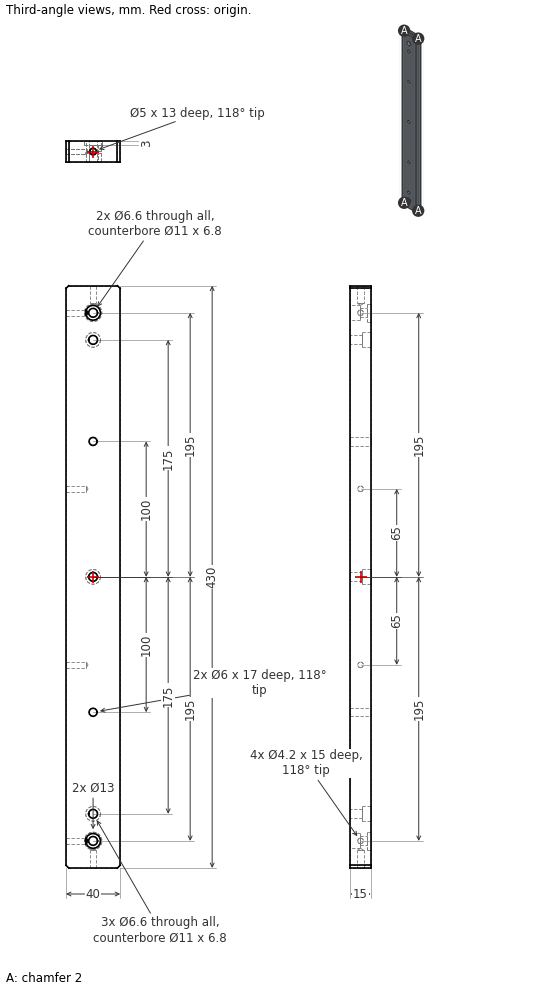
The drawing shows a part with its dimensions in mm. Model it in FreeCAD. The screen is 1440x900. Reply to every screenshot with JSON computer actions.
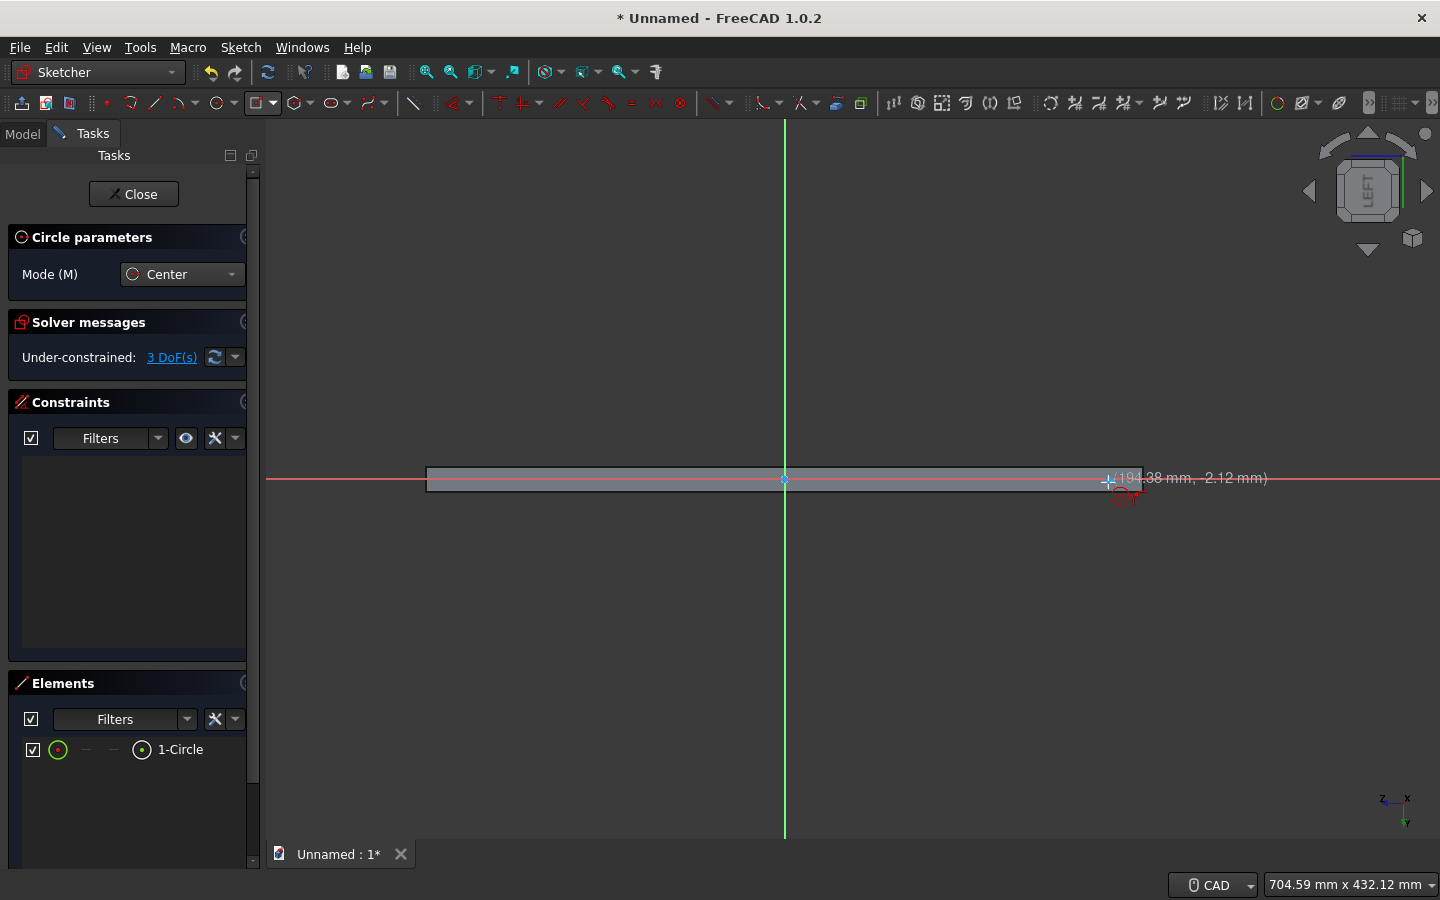
{"action": "scroll", "coordinate": [460, 479], "scroll_direction": "up", "scroll_amount": 10}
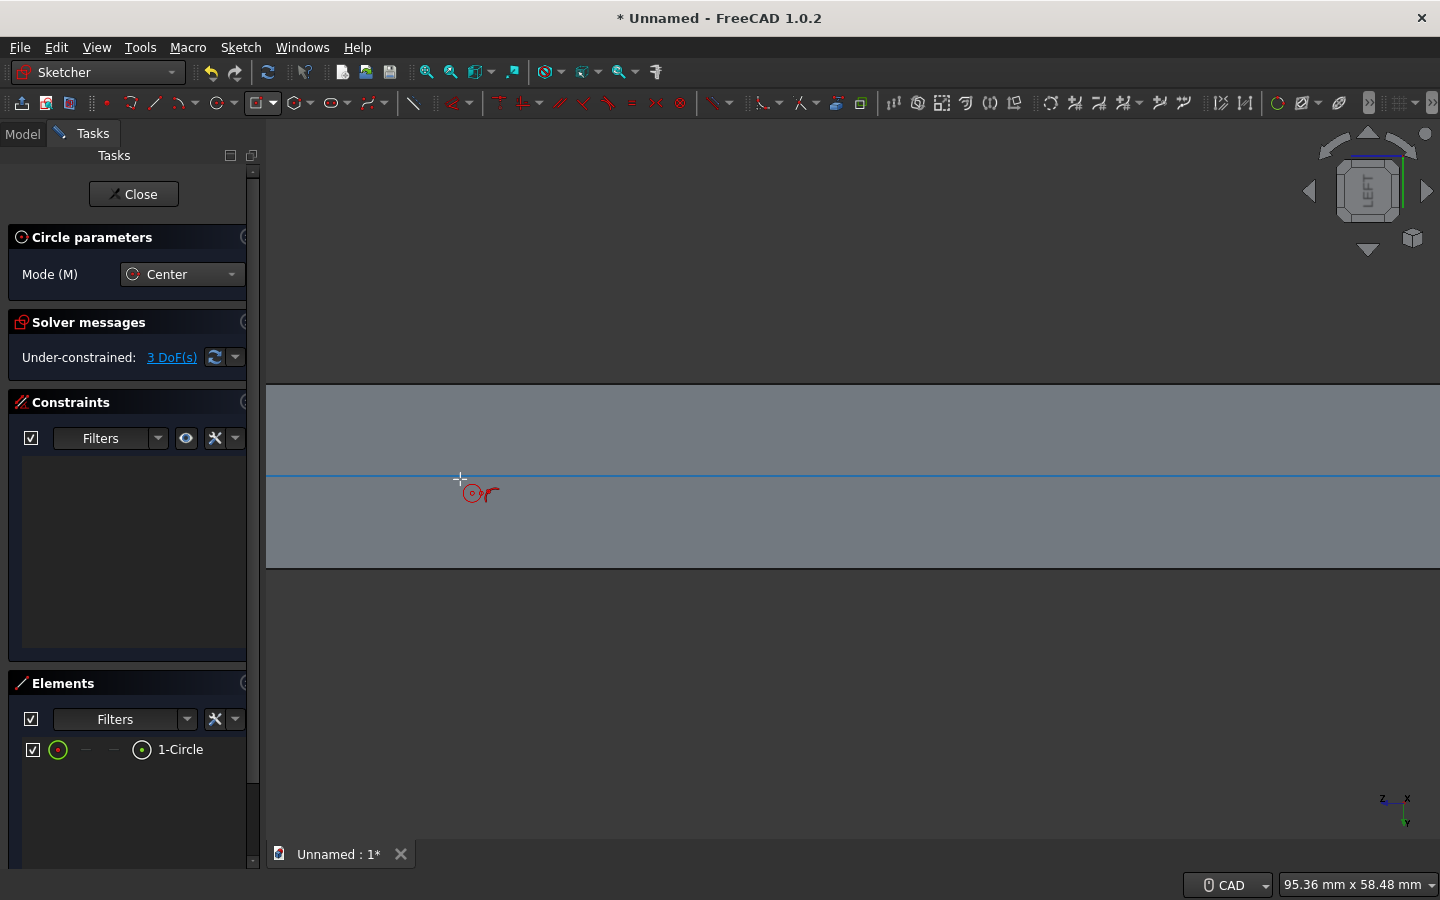
{"action": "scroll", "coordinate": [460, 479], "scroll_direction": "down", "scroll_amount": 10}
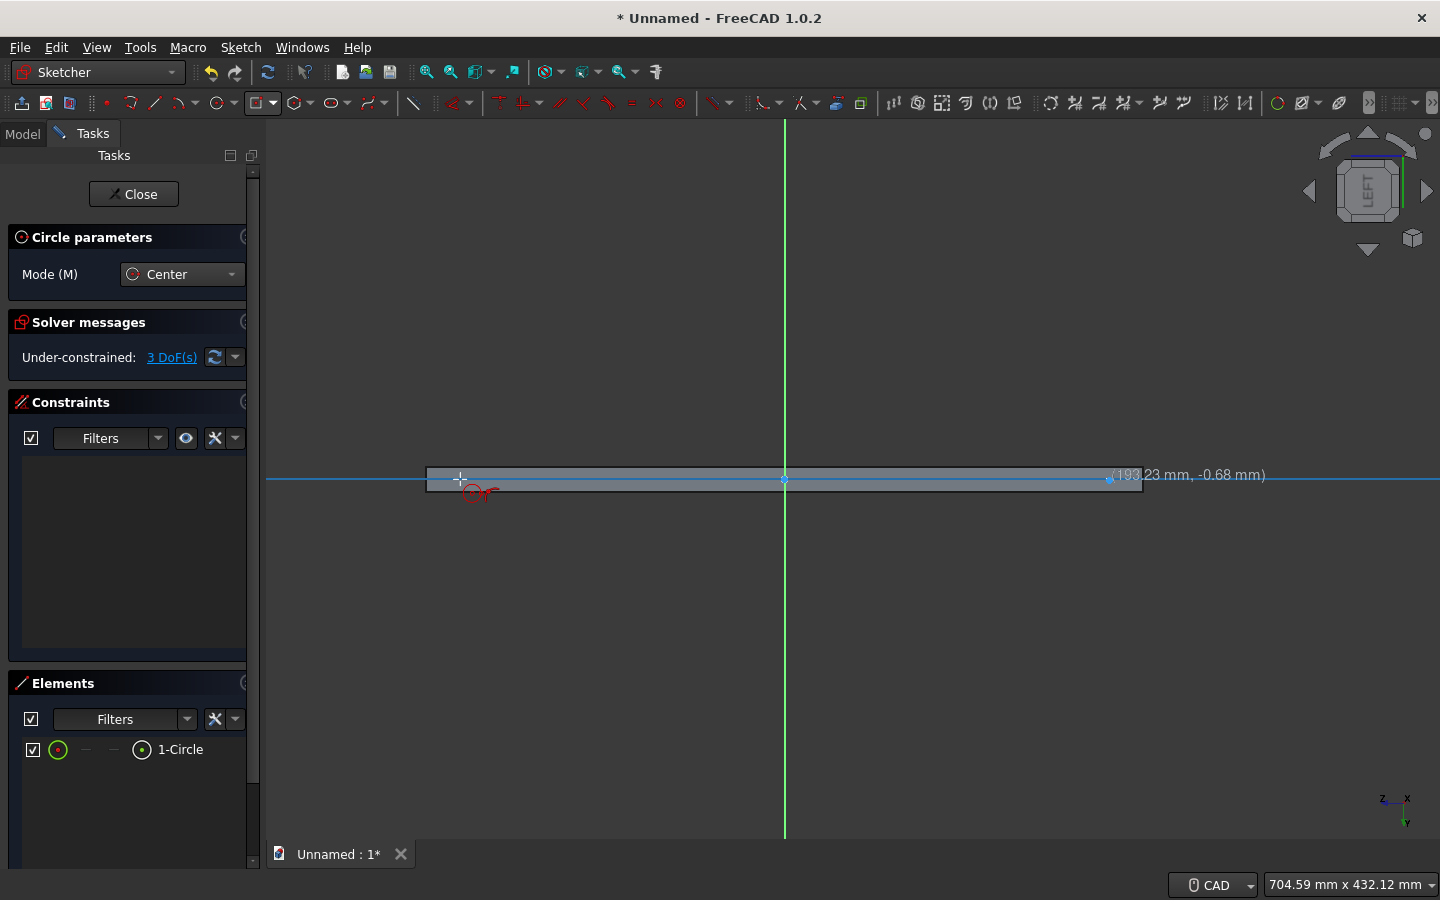
{"action": "left_click", "coordinate": [460, 479]}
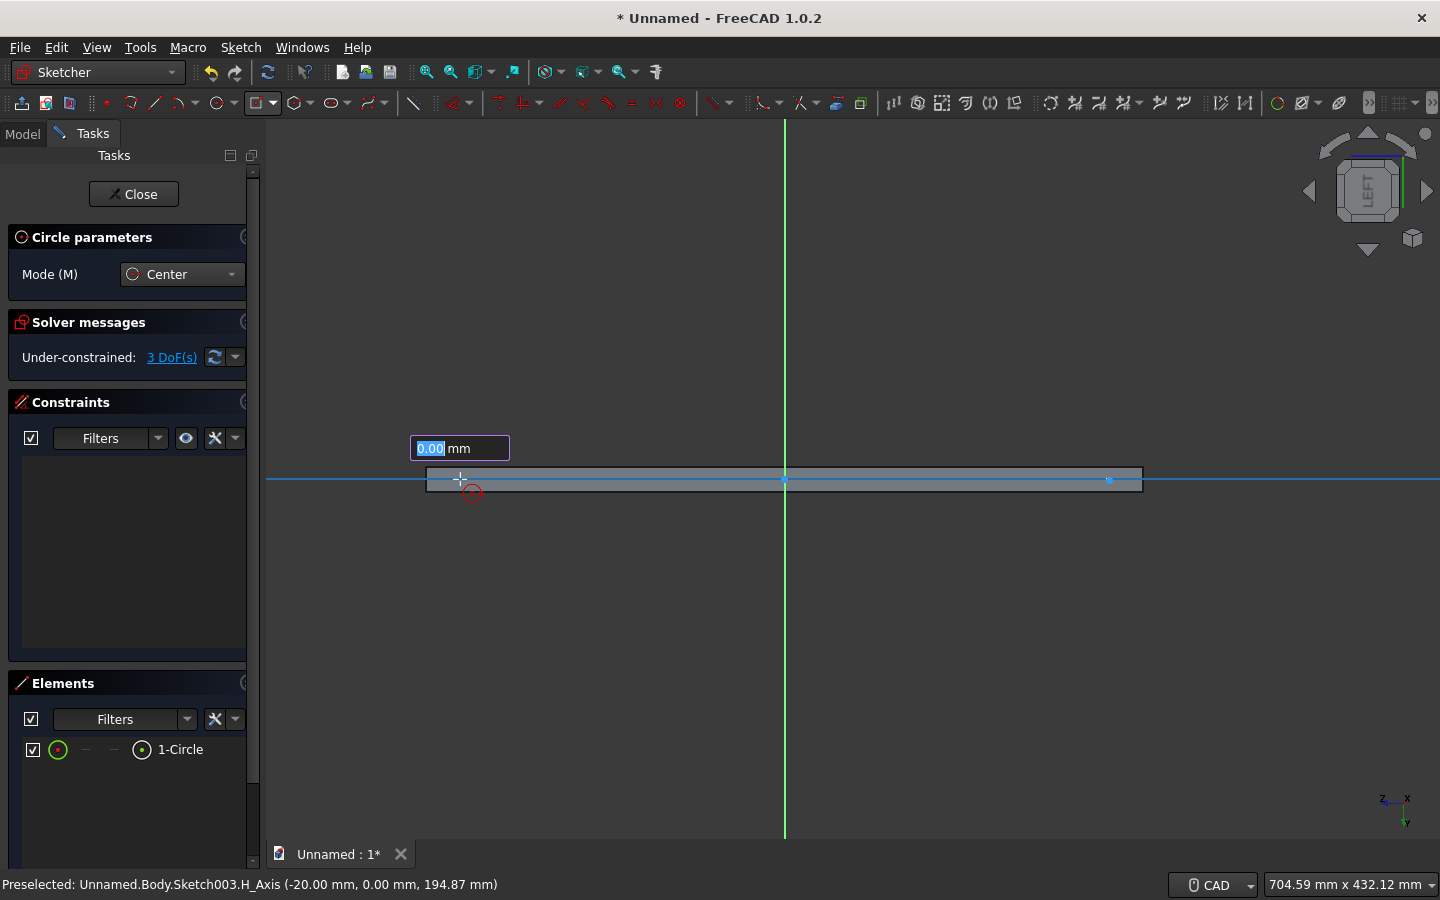
{"action": "scroll", "coordinate": [459, 482], "scroll_direction": "up", "scroll_amount": 8}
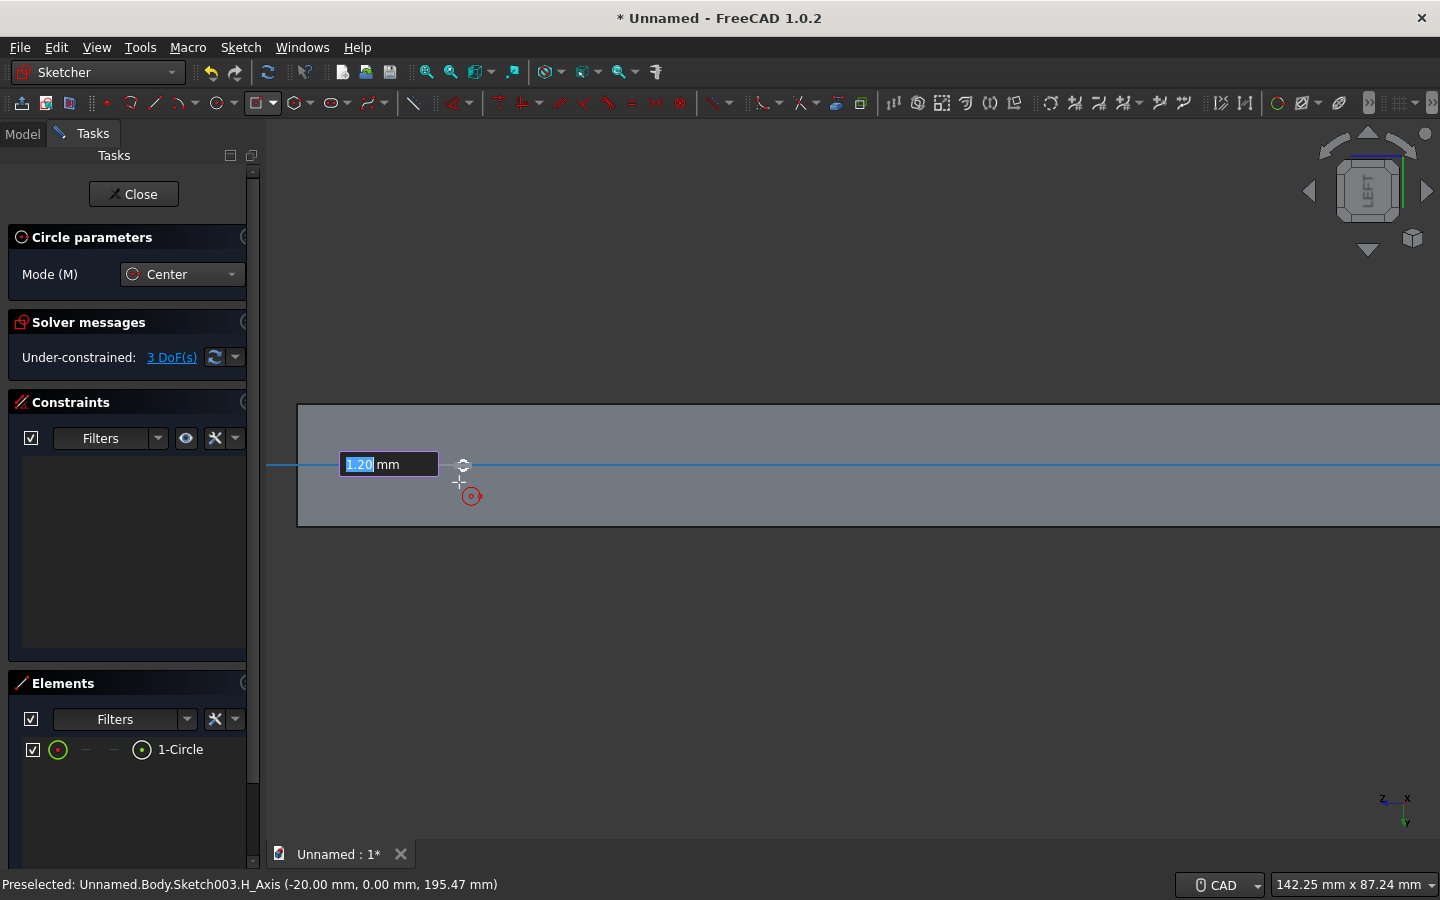
{"action": "left_click", "coordinate": [456, 482]}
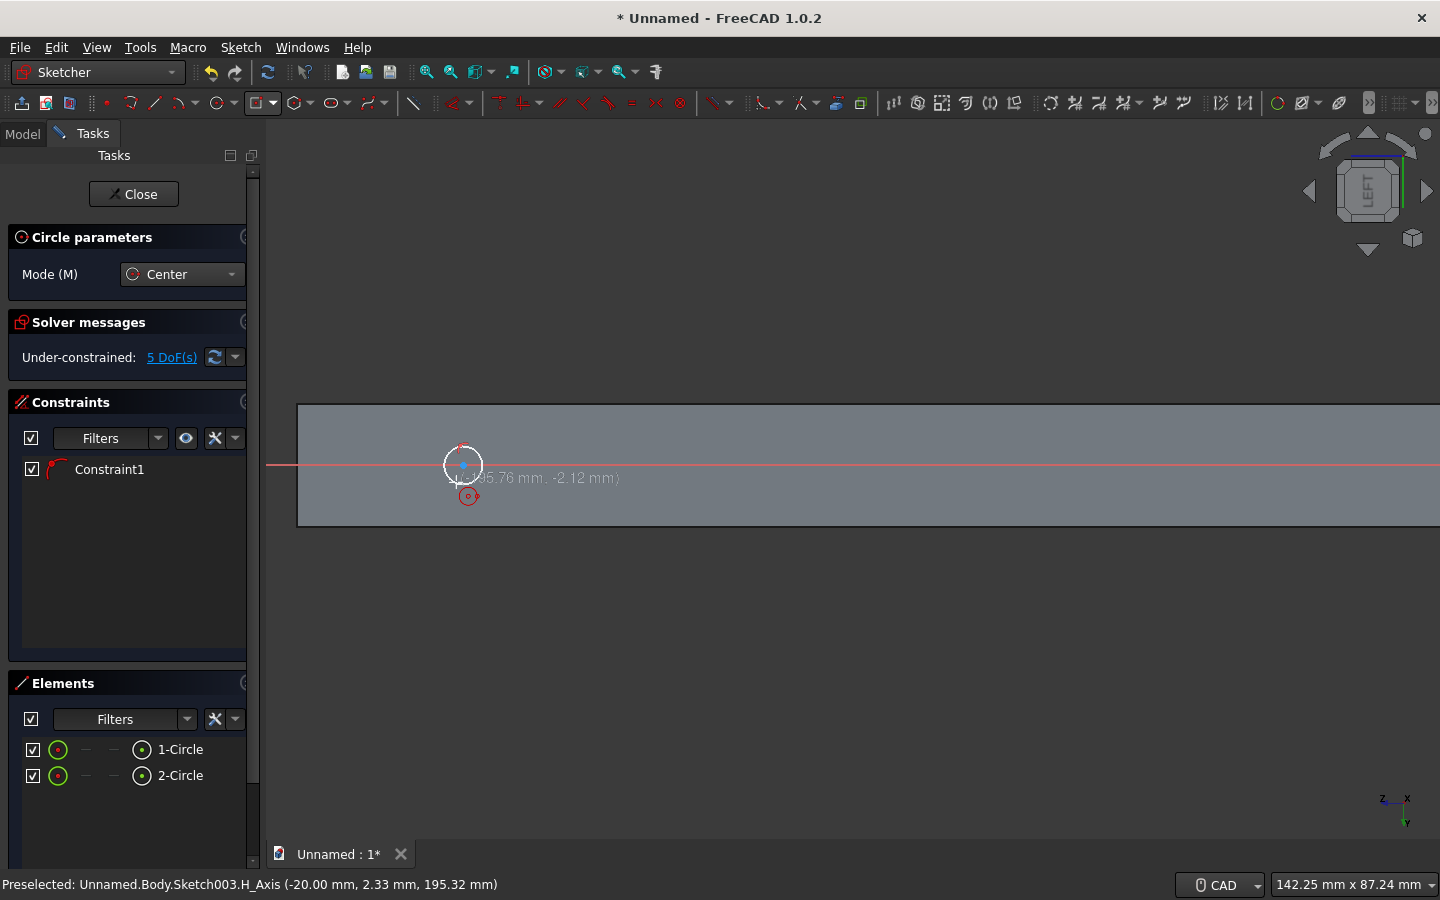
{"action": "scroll", "coordinate": [459, 482], "scroll_direction": "down", "scroll_amount": 8}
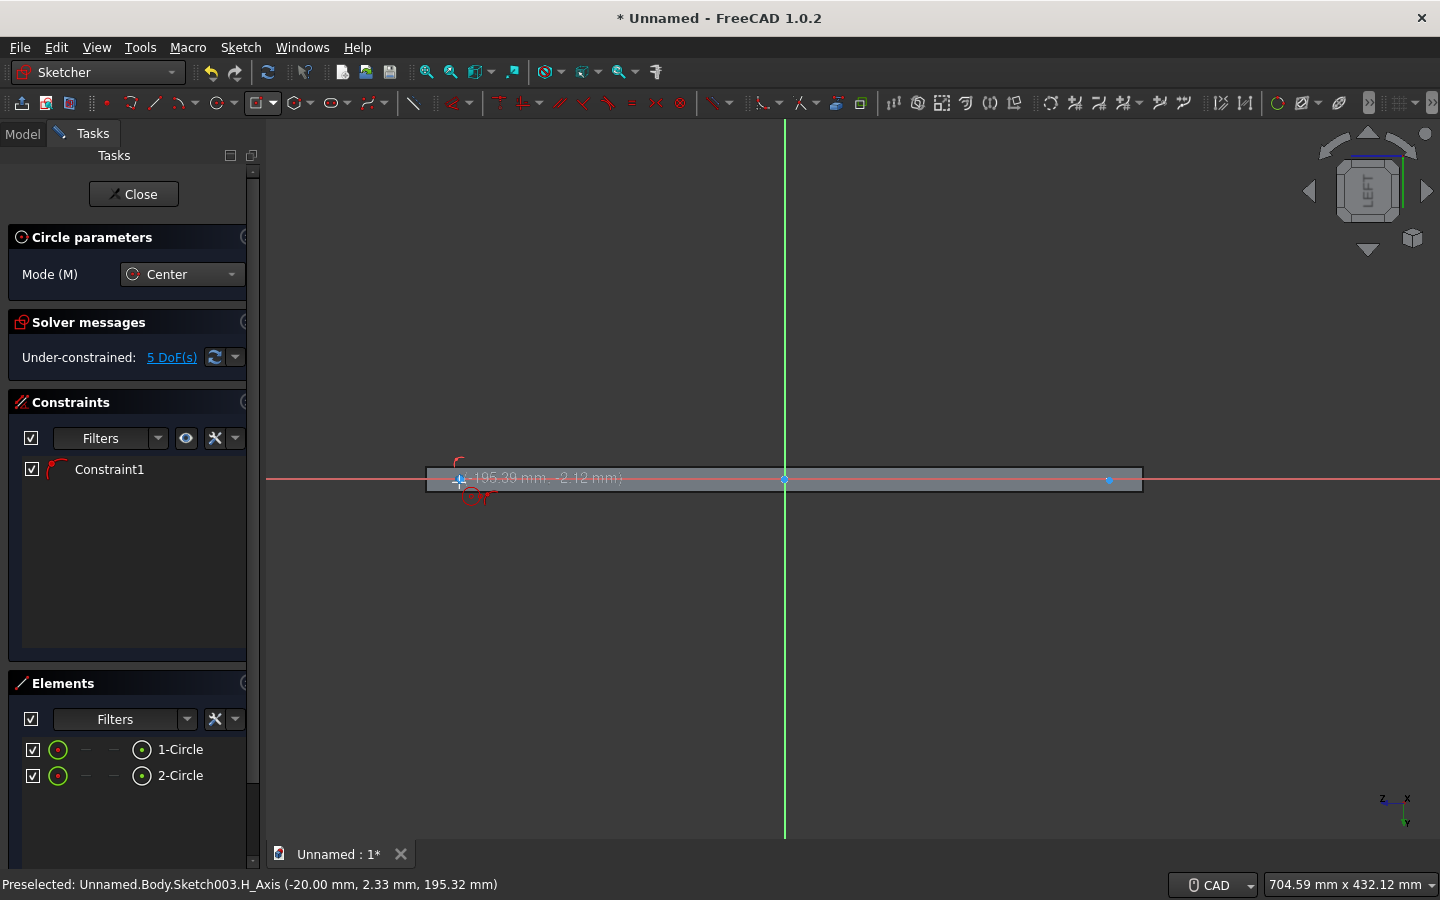
{"action": "scroll", "coordinate": [893, 479], "scroll_direction": "up", "scroll_amount": 10}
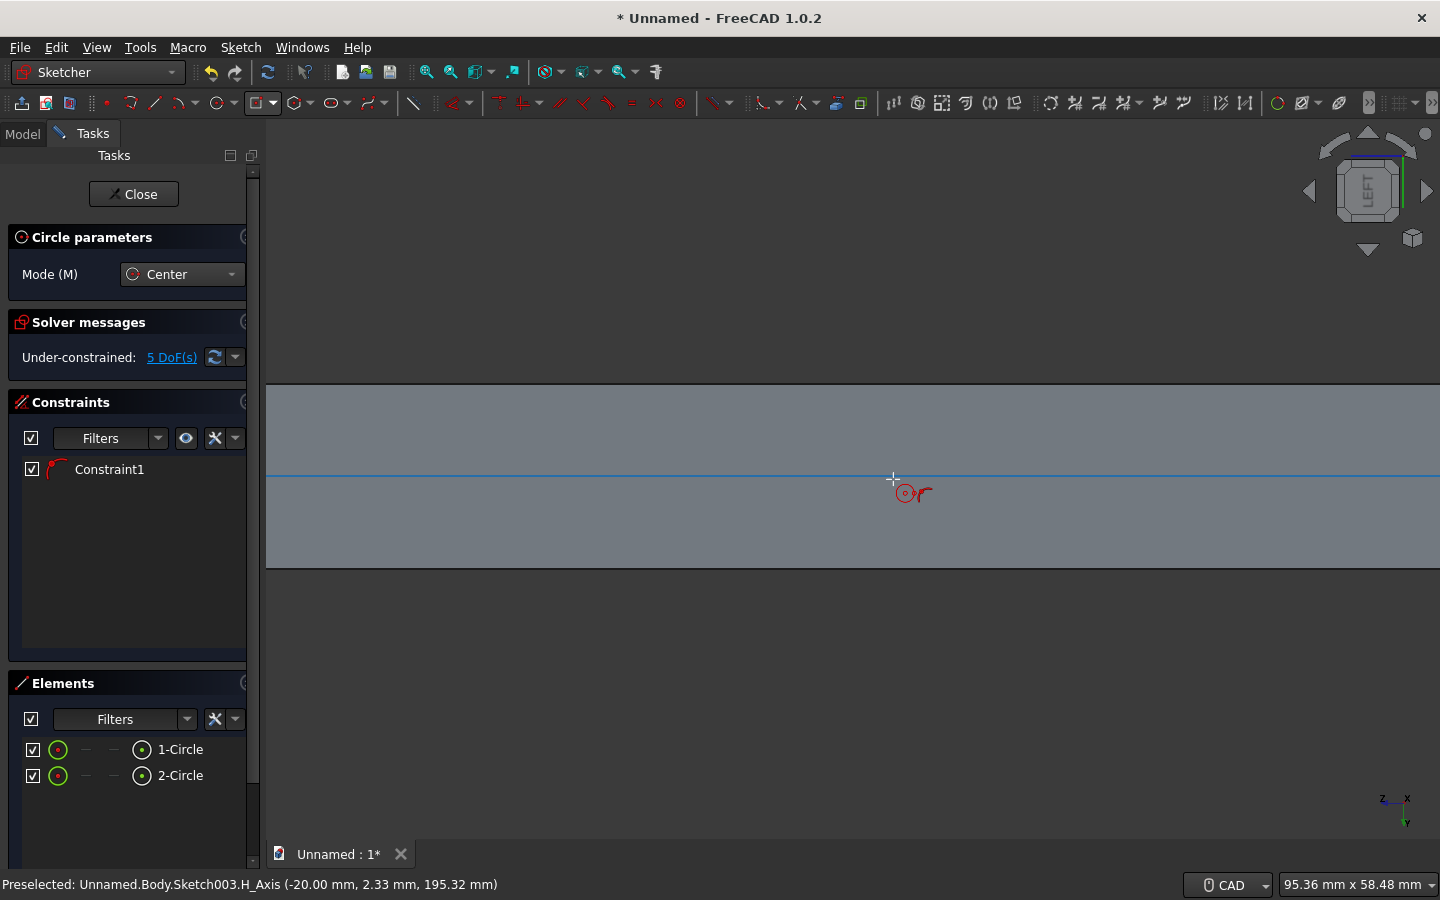
{"action": "scroll", "coordinate": [893, 479], "scroll_direction": "down", "scroll_amount": 10}